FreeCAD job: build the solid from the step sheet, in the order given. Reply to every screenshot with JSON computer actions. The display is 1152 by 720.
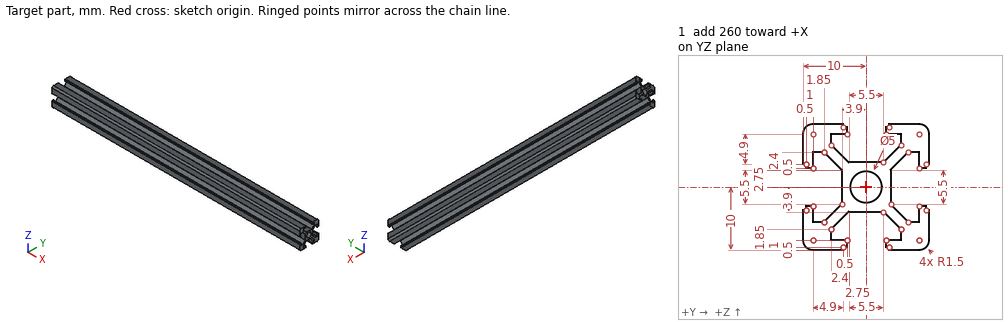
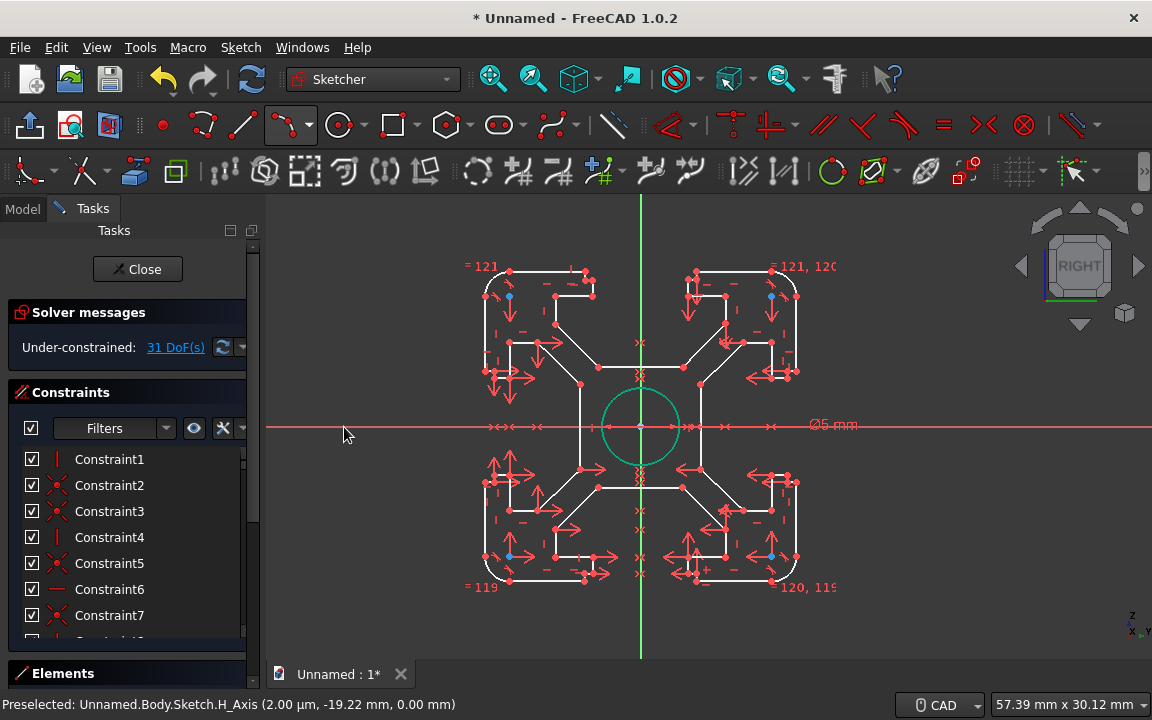
{"action": "left_click", "coordinate": [683, 488]}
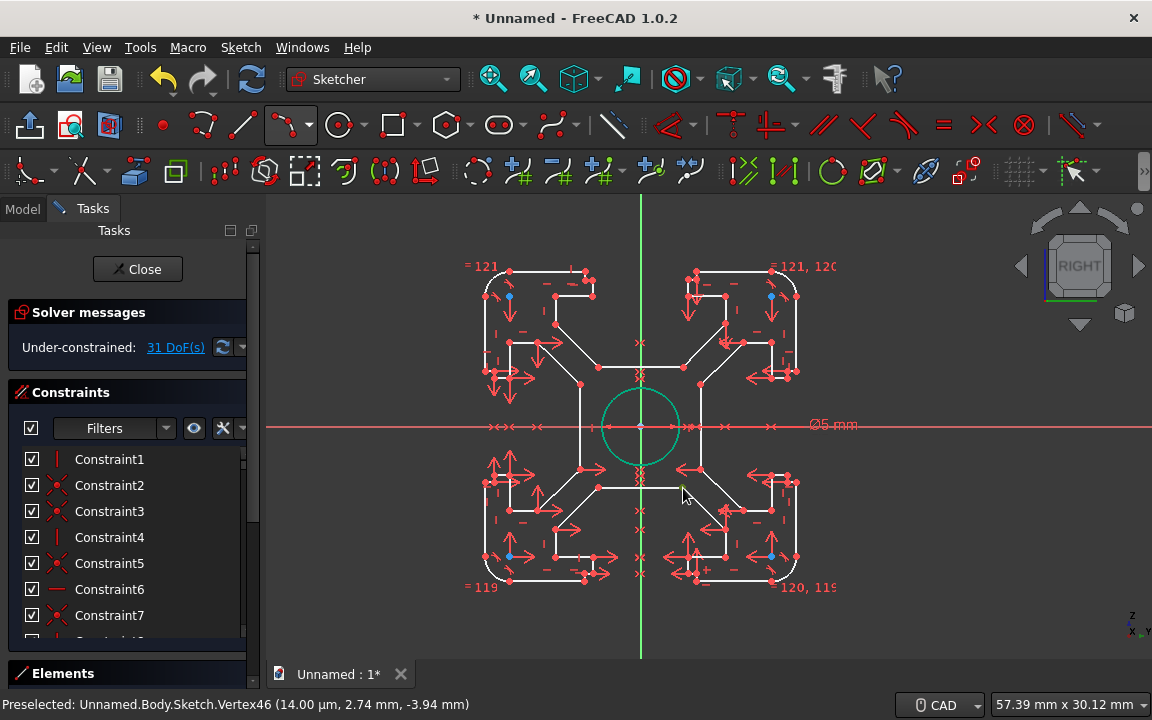
{"action": "left_click", "coordinate": [683, 367]}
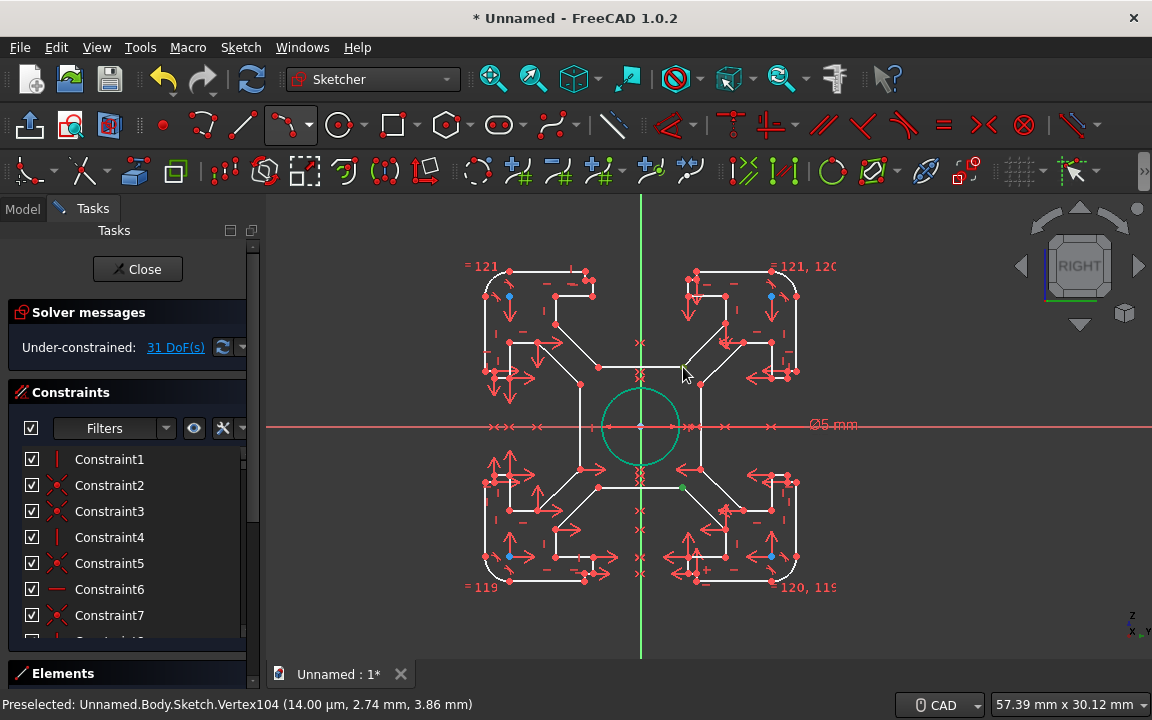
{"action": "left_click", "coordinate": [344, 427]}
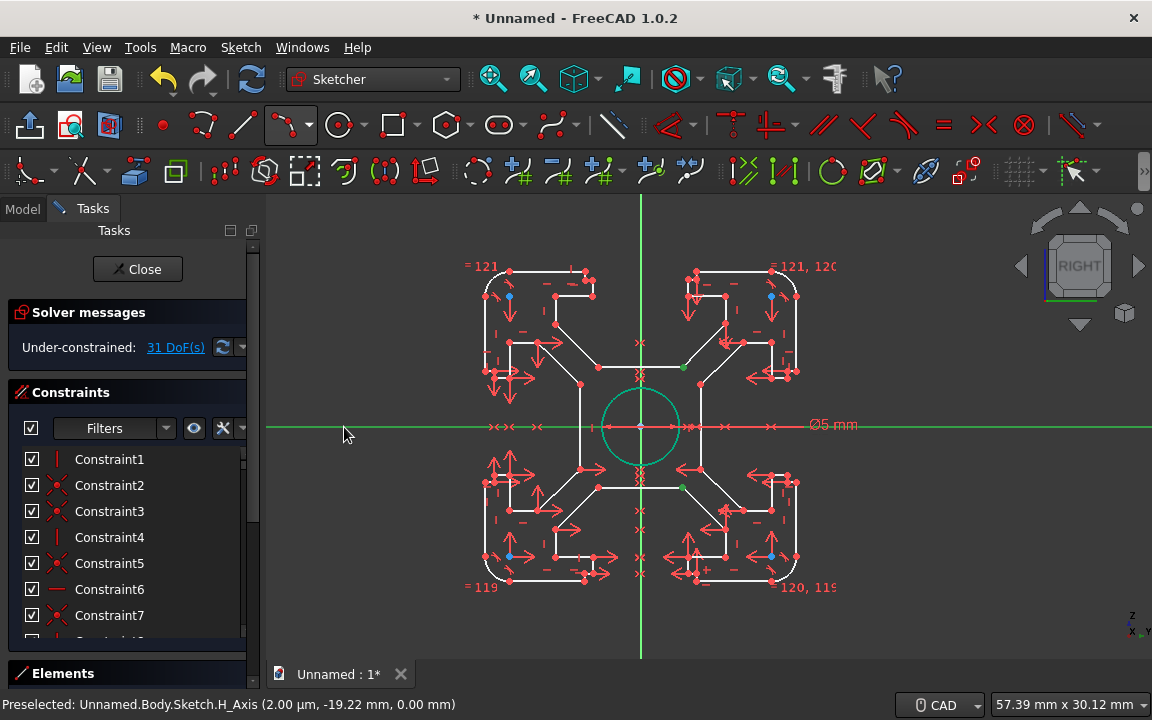
{"action": "left_click", "coordinate": [984, 126]}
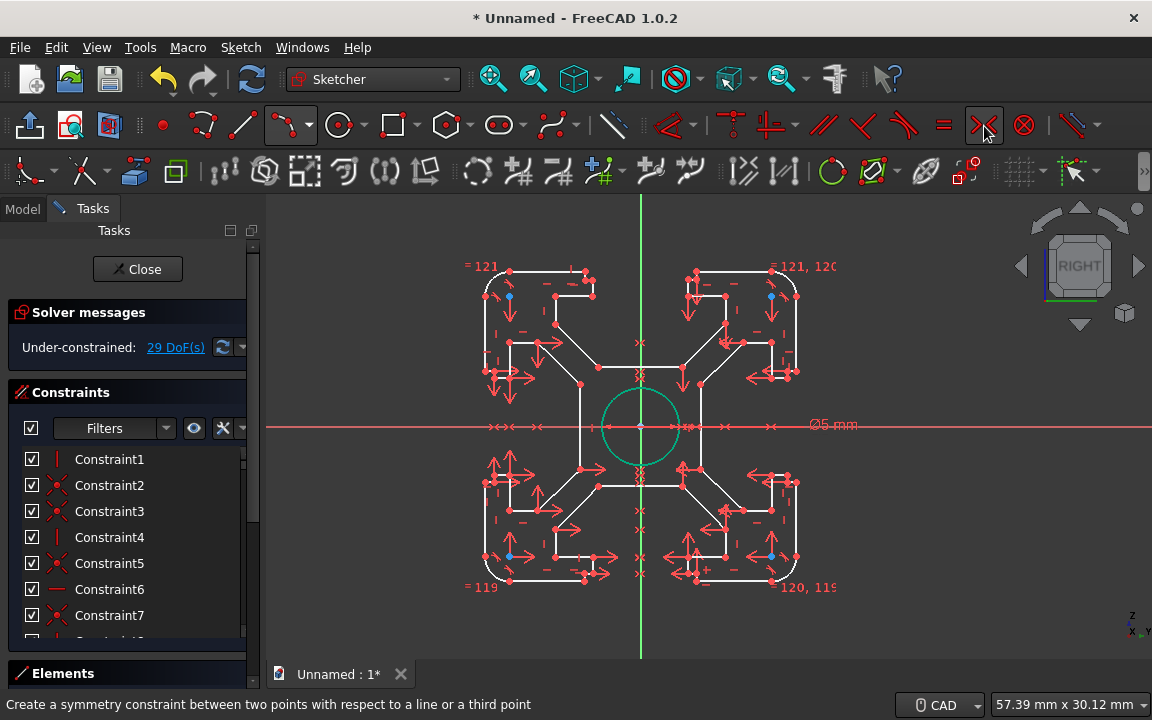
{"action": "left_click", "coordinate": [556, 530]}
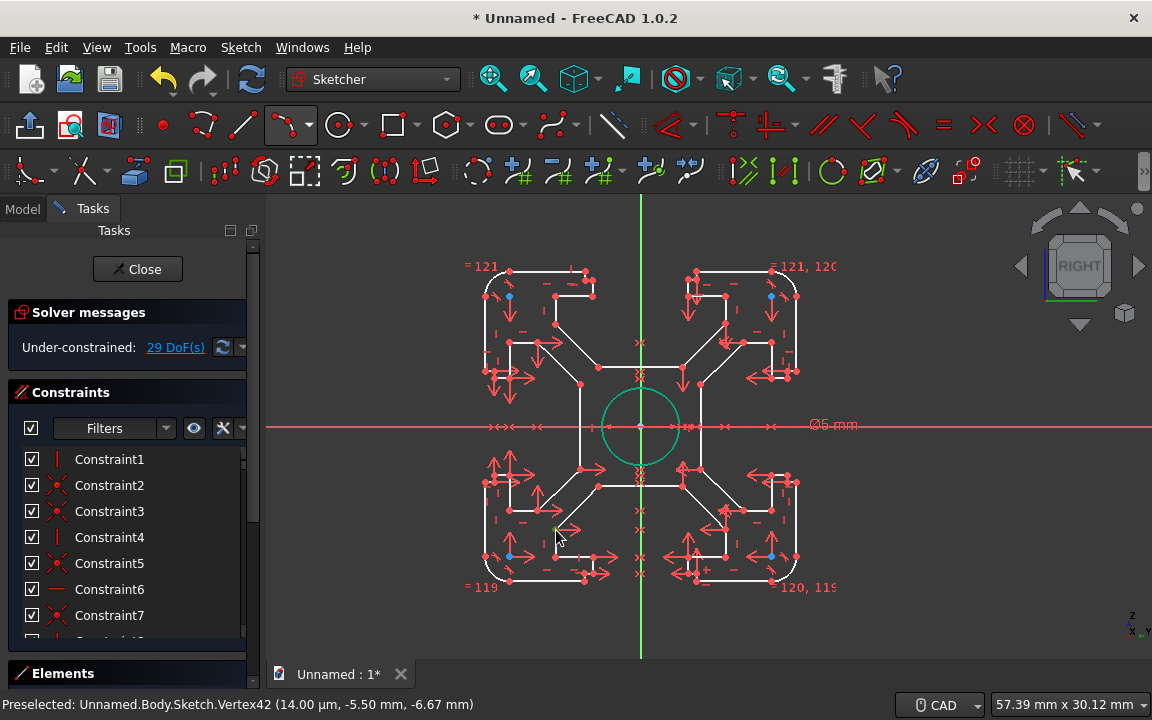
{"action": "left_click", "coordinate": [556, 324]}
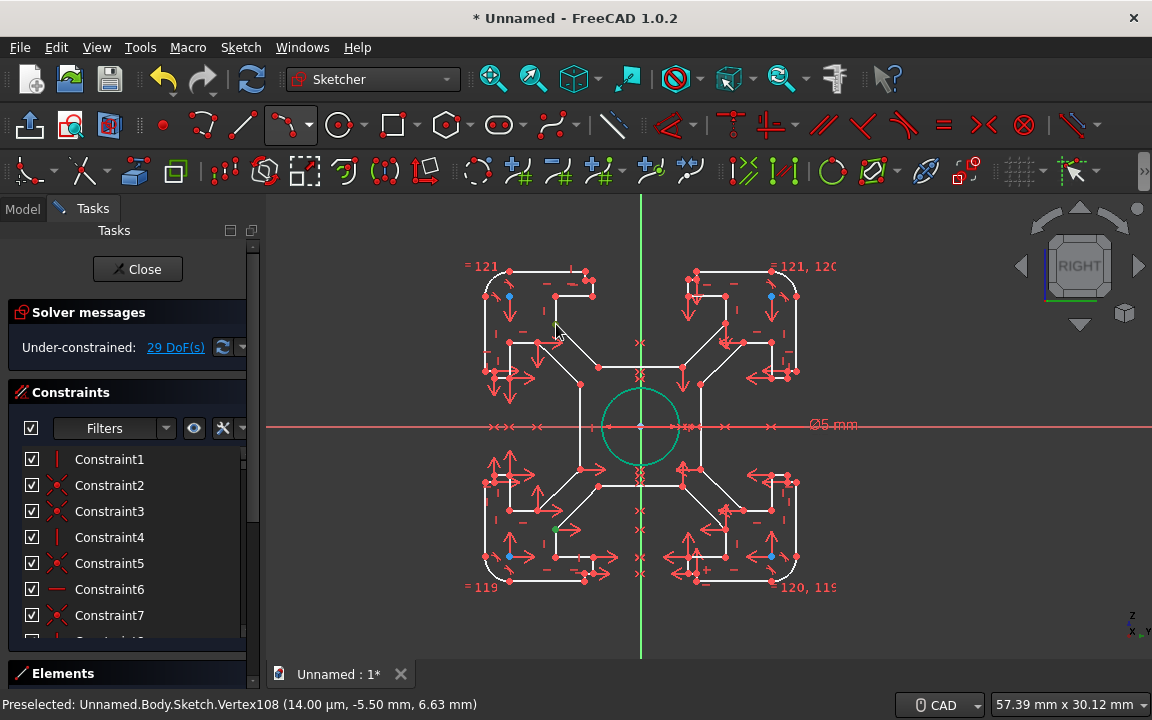
{"action": "left_click", "coordinate": [344, 427]}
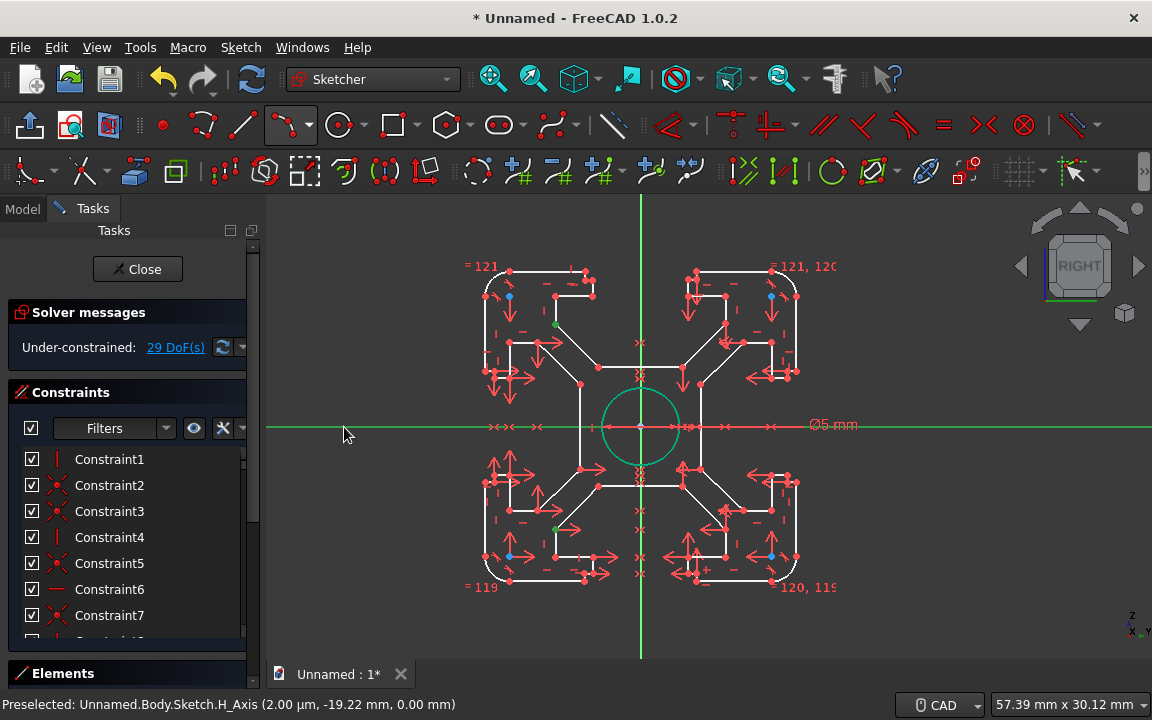
{"action": "left_click", "coordinate": [984, 126]}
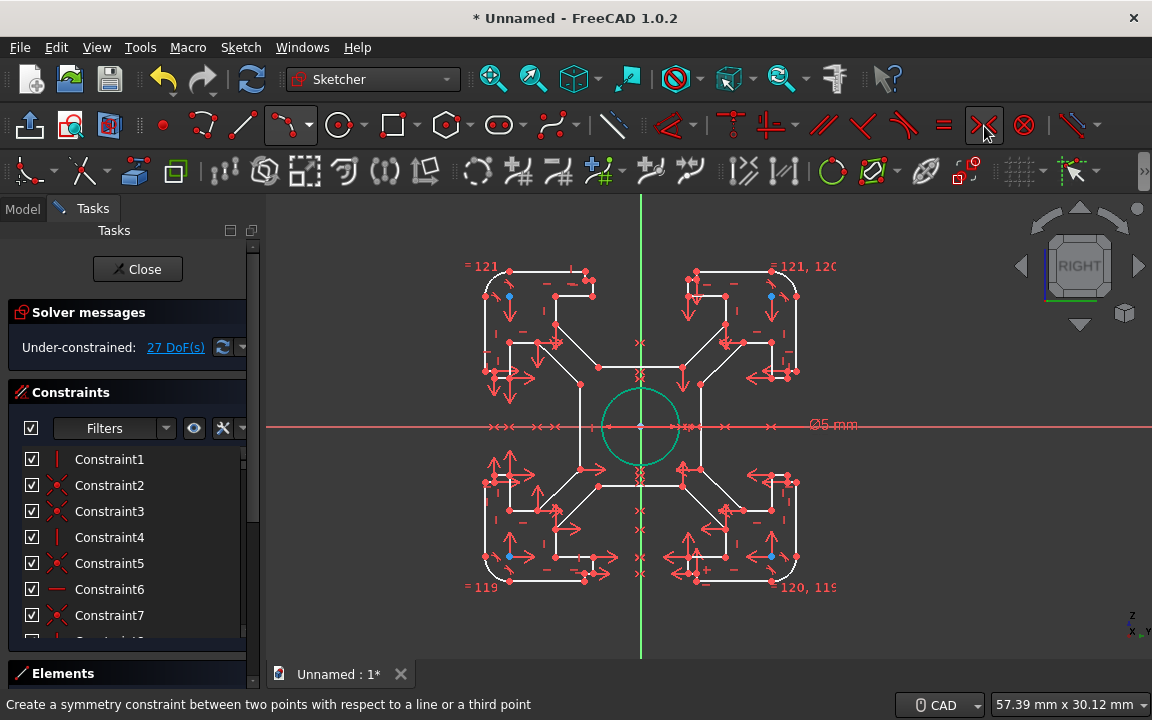
{"action": "left_click", "coordinate": [593, 557]}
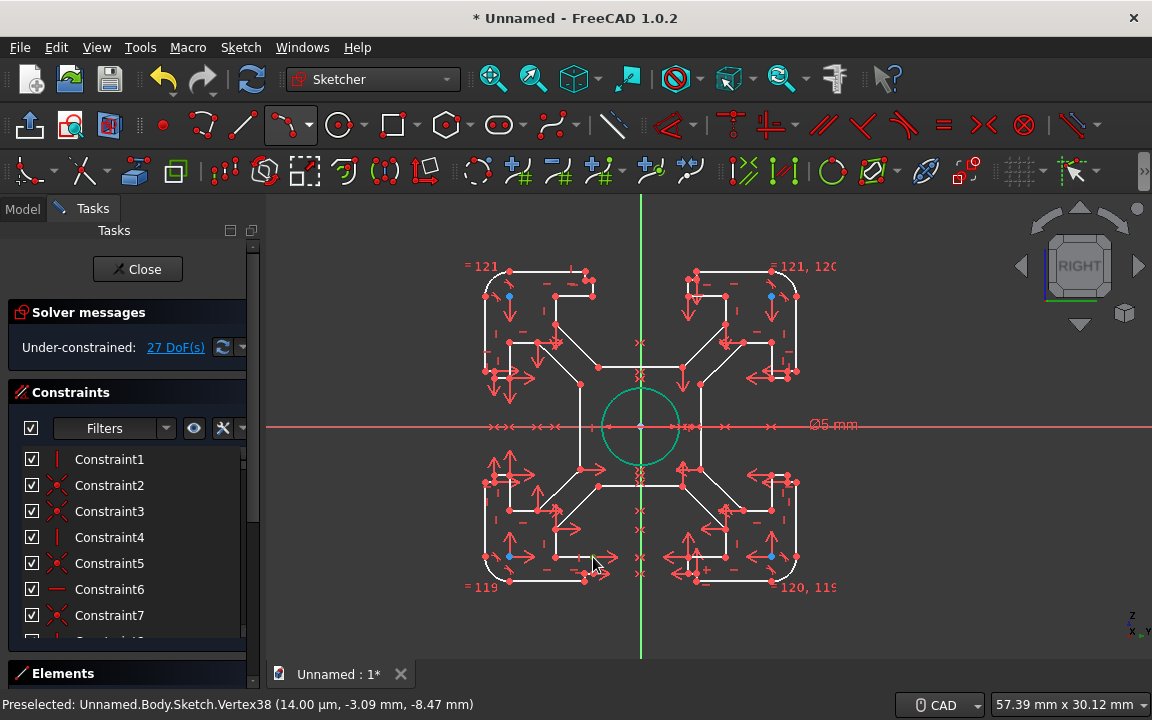
{"action": "left_click", "coordinate": [593, 296]}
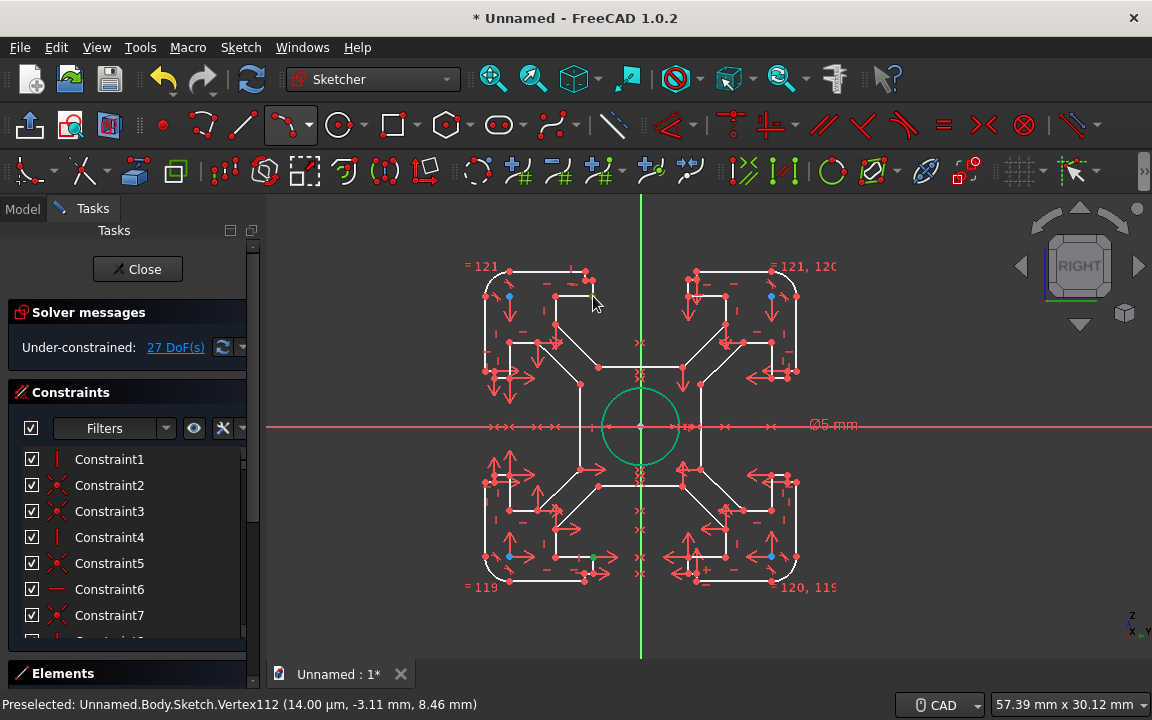
{"action": "left_click", "coordinate": [344, 427]}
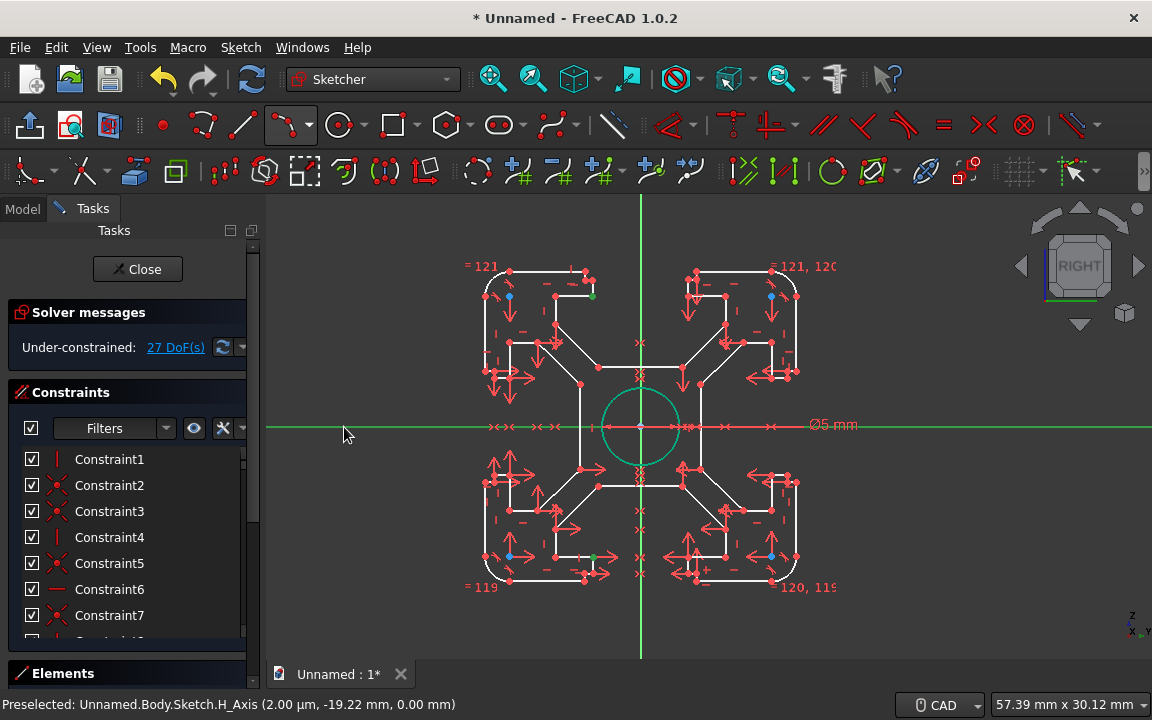
{"action": "left_click", "coordinate": [984, 126]}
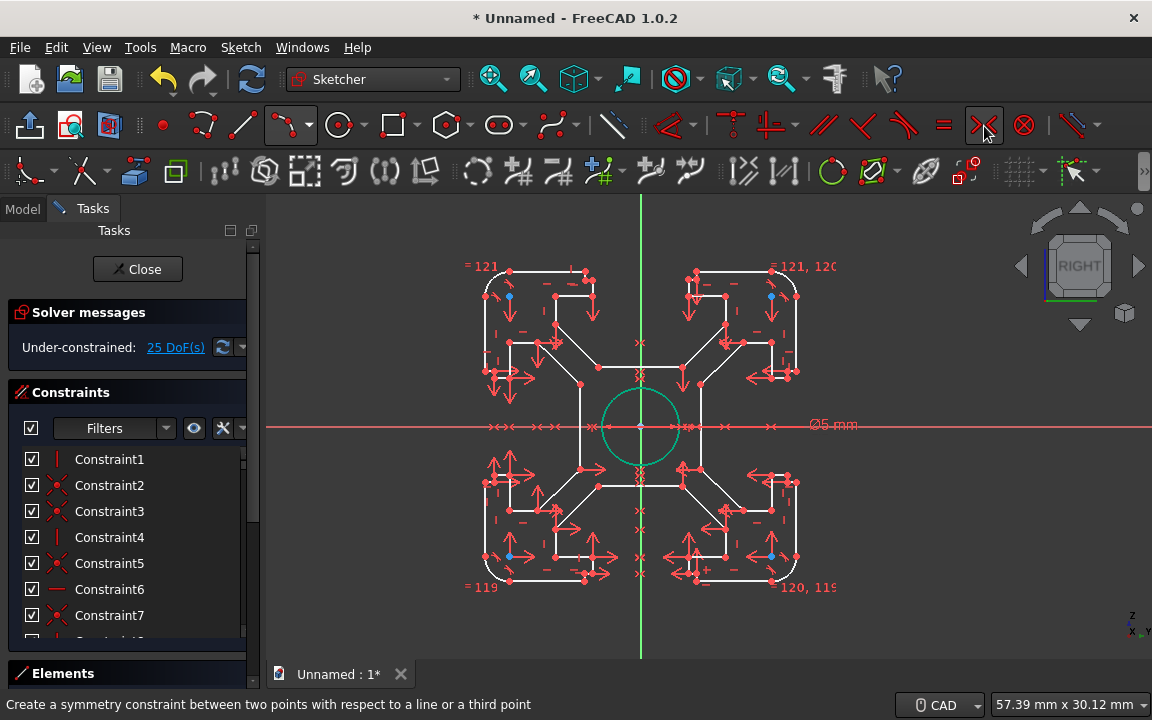
{"action": "scroll", "coordinate": [585, 574], "scroll_direction": "up", "scroll_amount": 3}